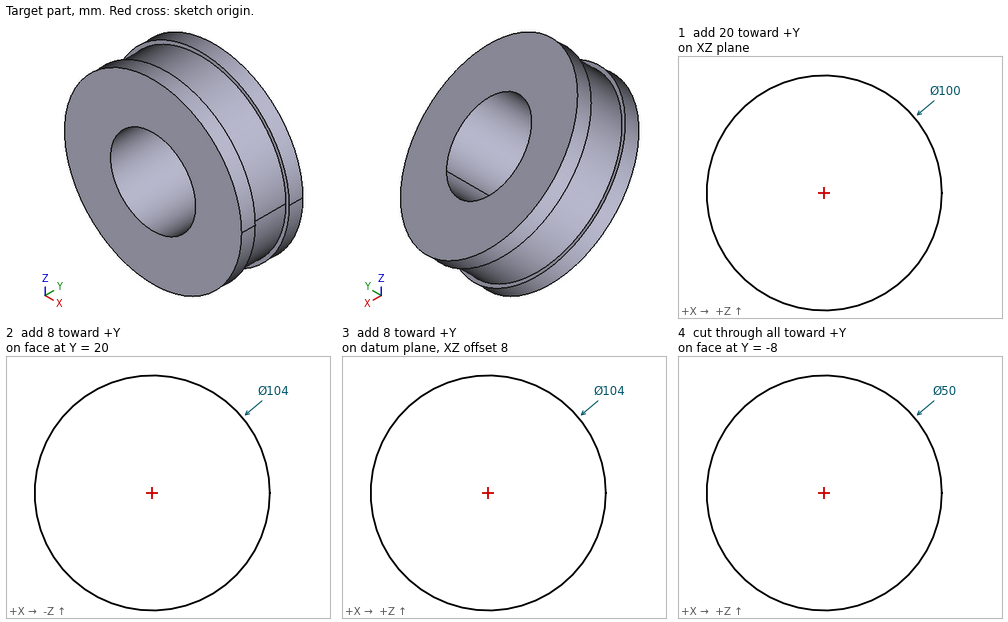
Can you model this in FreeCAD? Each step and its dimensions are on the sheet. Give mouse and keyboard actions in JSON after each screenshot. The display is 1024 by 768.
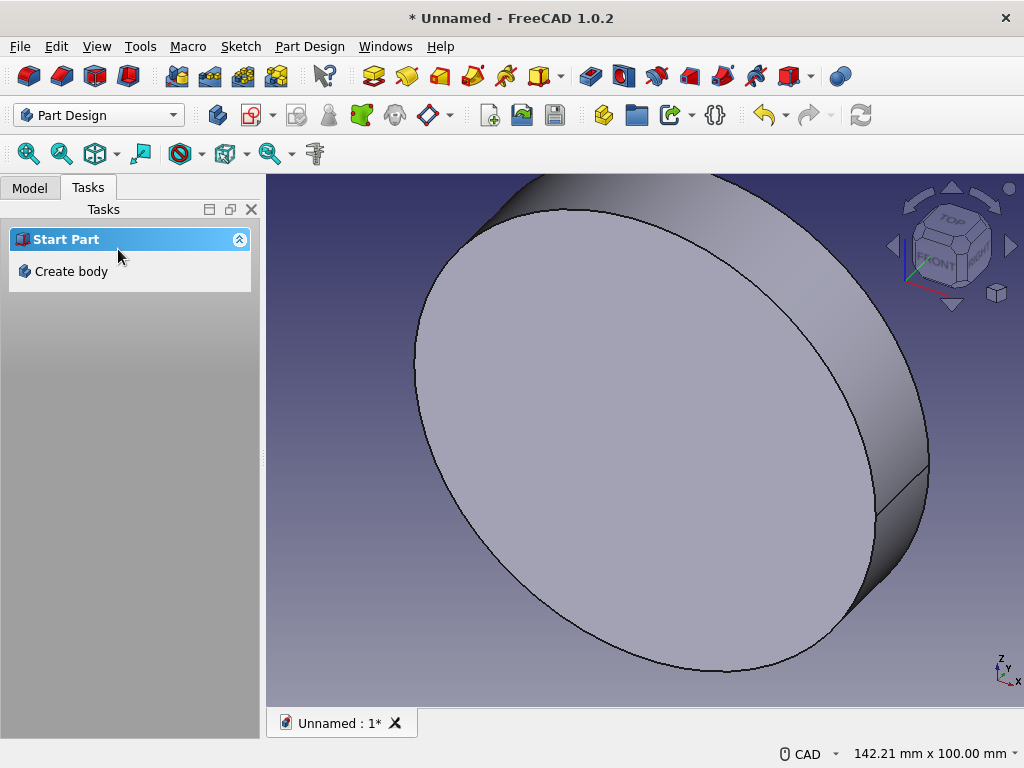
{"action": "left_click", "coordinate": [29, 154]}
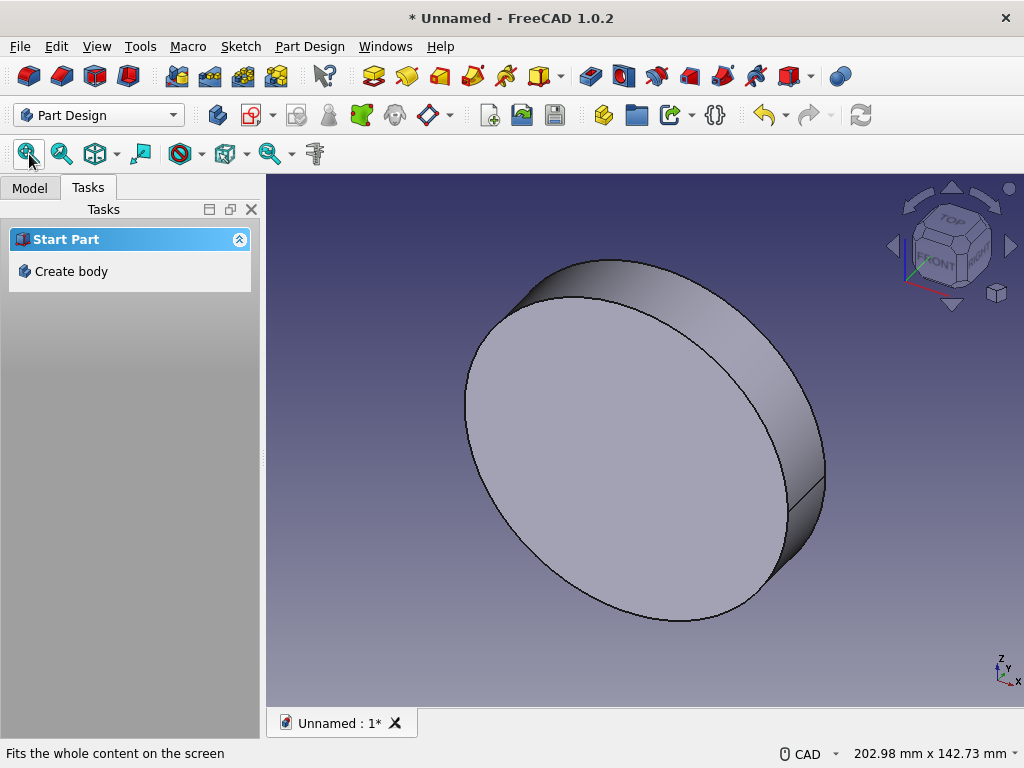
{"action": "key", "text": "4"}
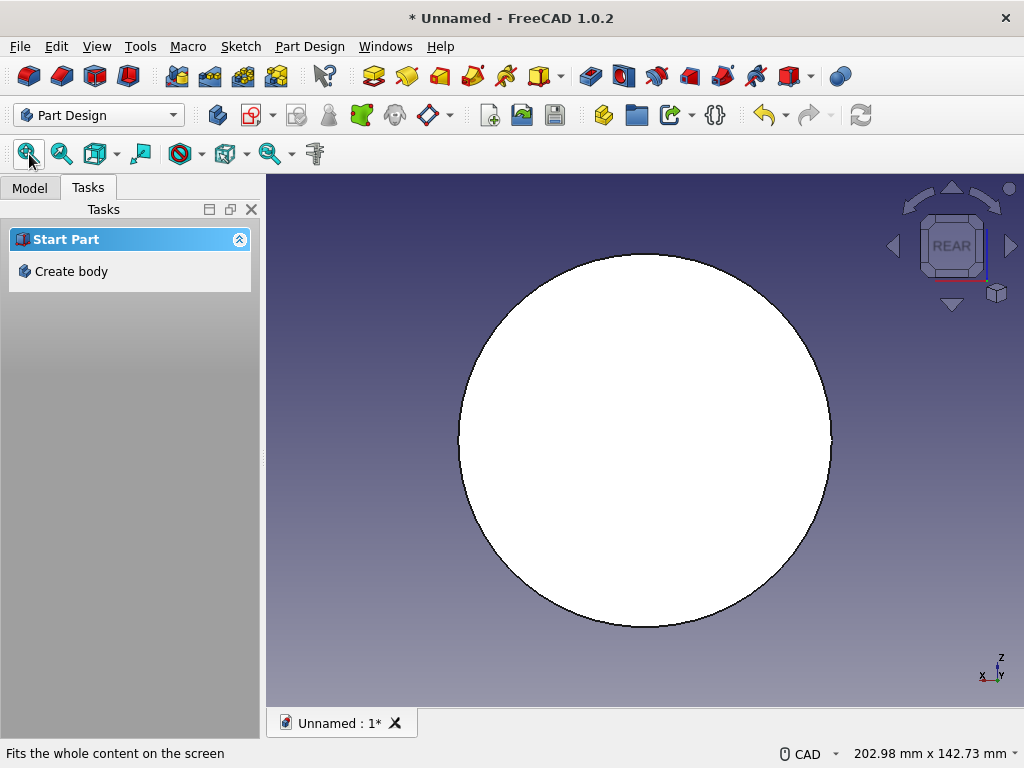
{"action": "left_click", "coordinate": [645, 440]}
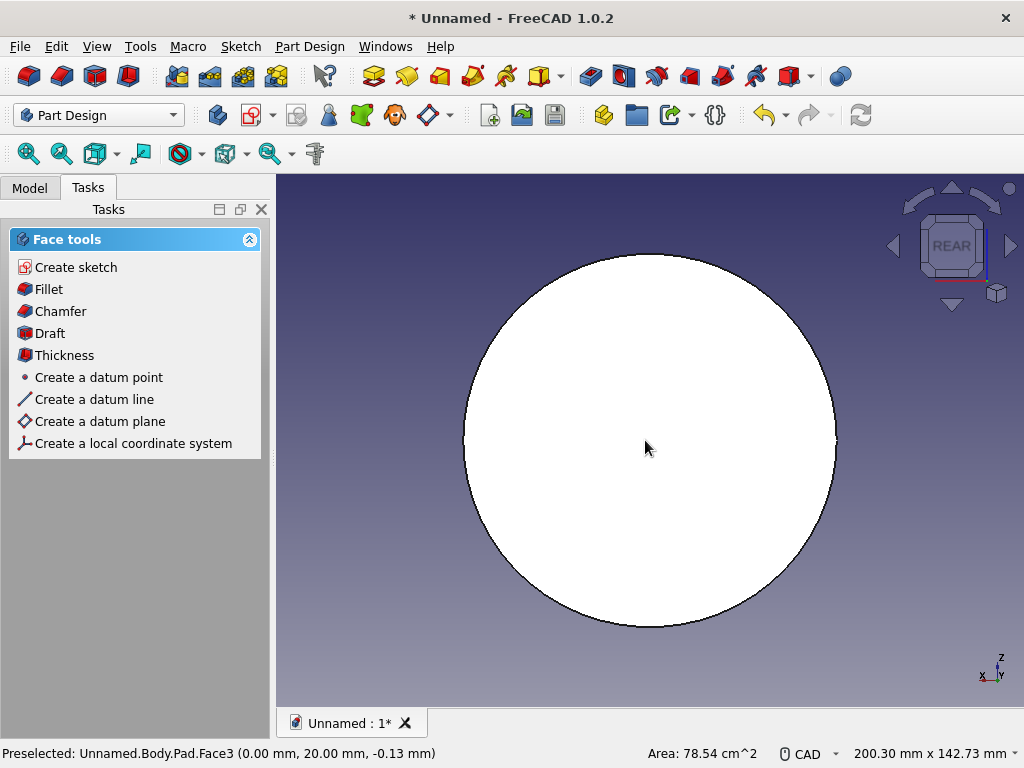
{"action": "left_click", "coordinate": [250, 116]}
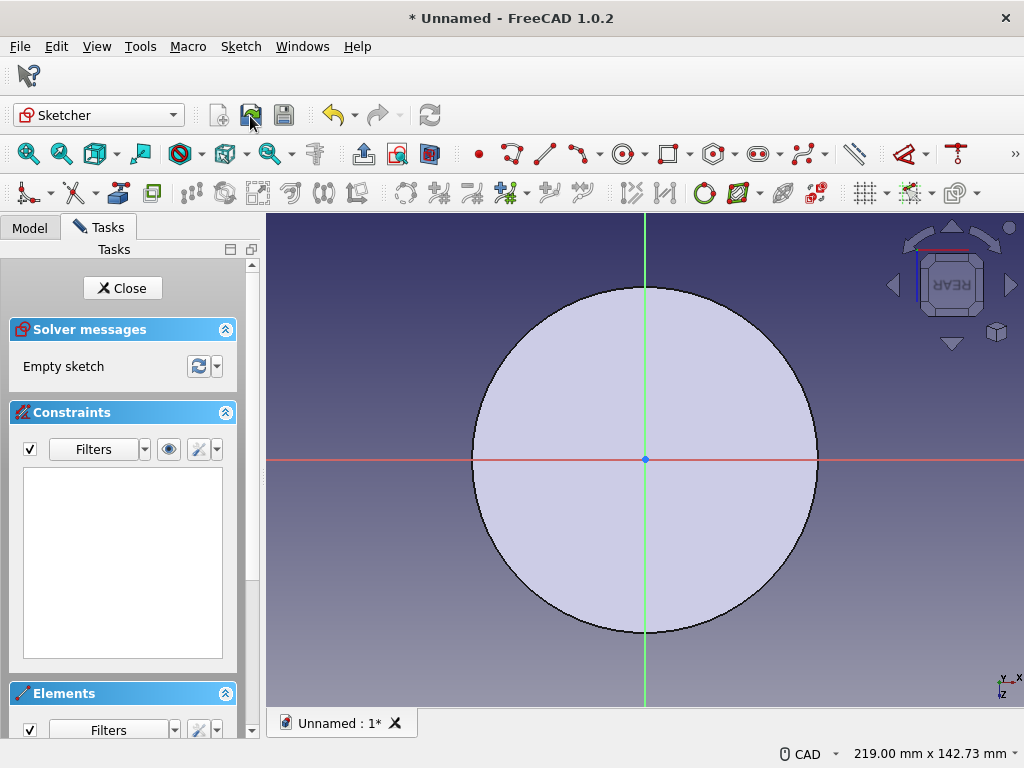
{"action": "left_click", "coordinate": [622, 154]}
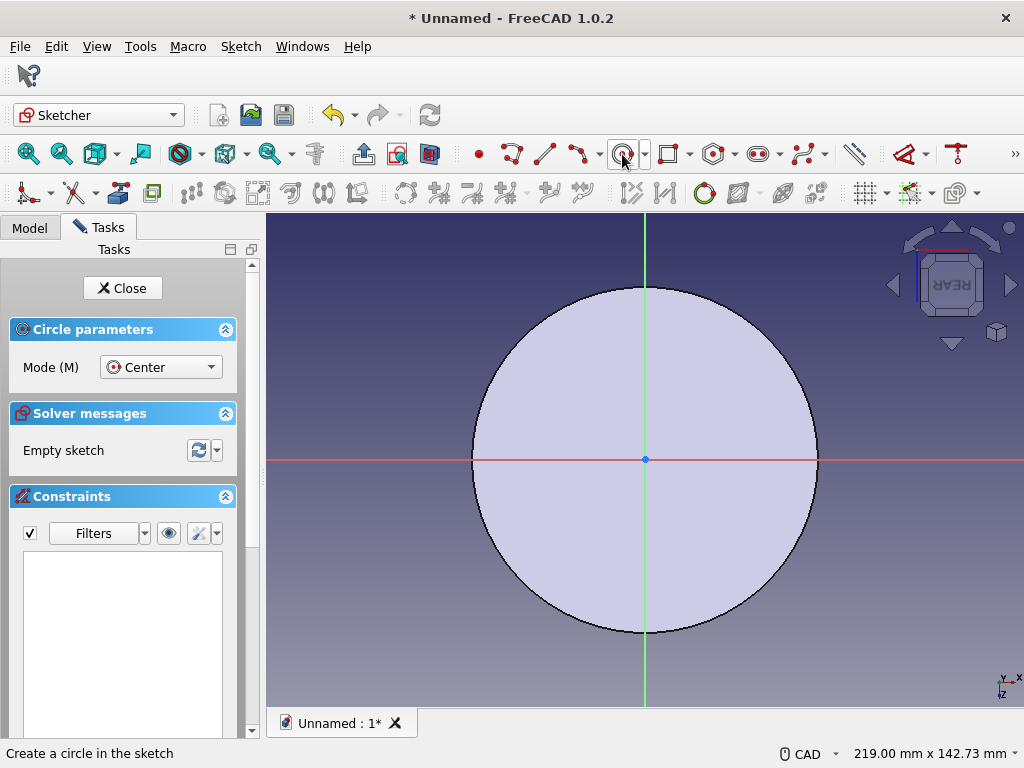
{"action": "left_click", "coordinate": [645, 460]}
{"action": "mouse_move", "coordinate": [772, 333]}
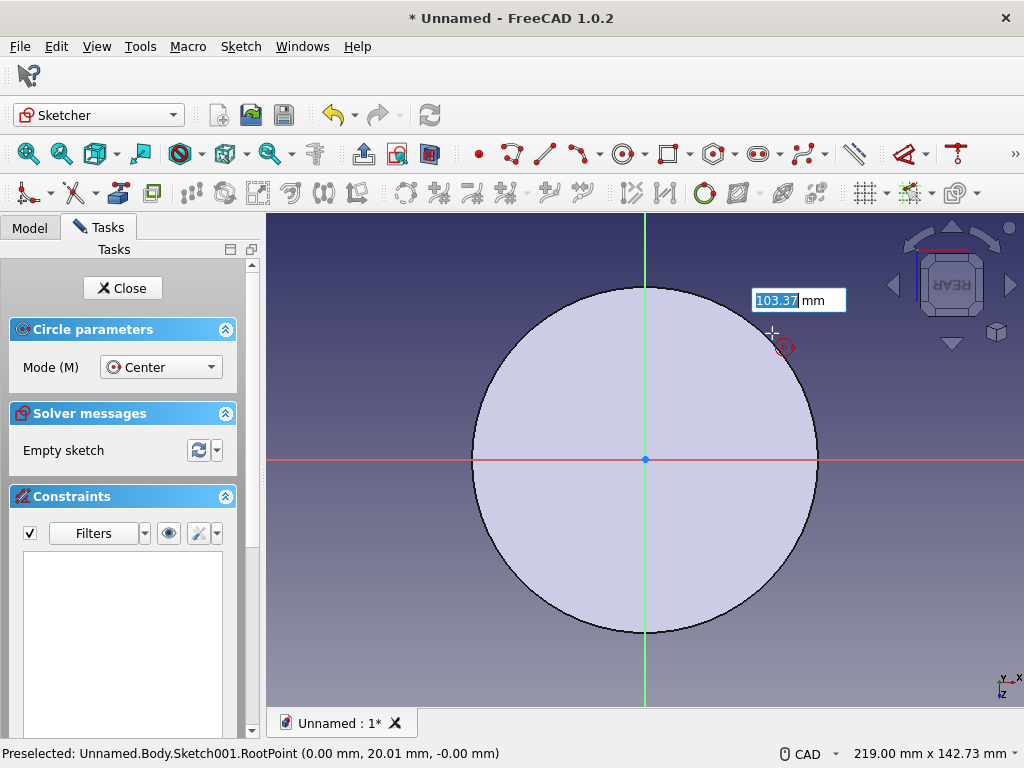
{"action": "type", "text": "104"}
{"action": "key", "text": "Return"}
{"action": "key", "text": "Escape"}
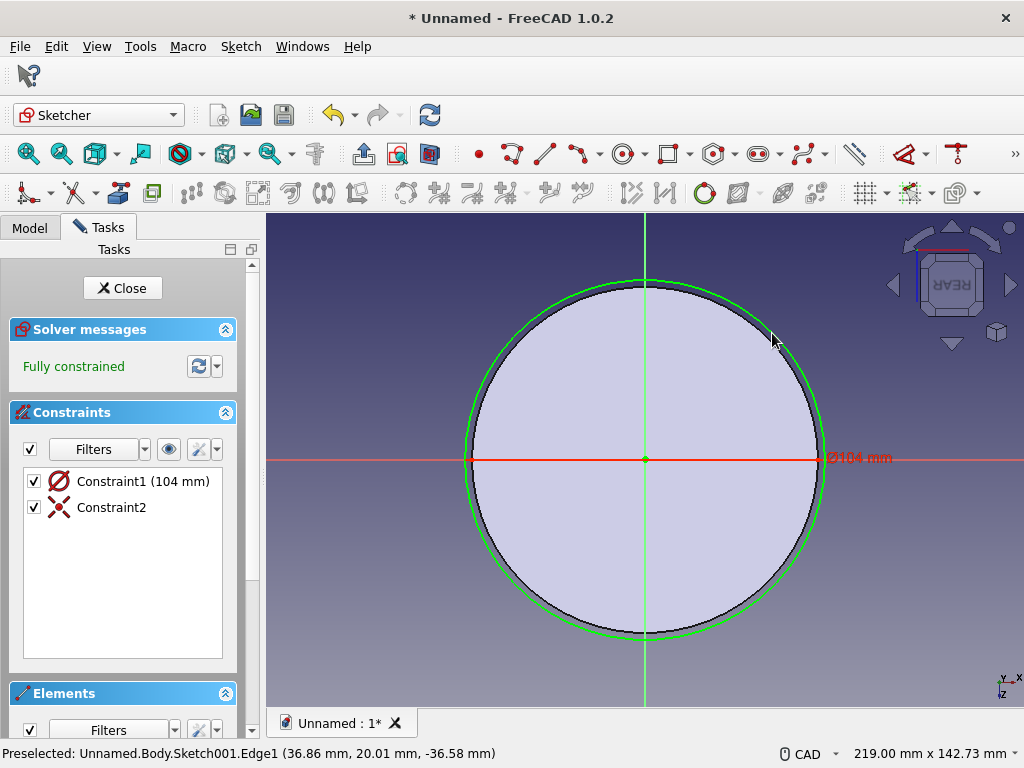
{"action": "left_click", "coordinate": [123, 288]}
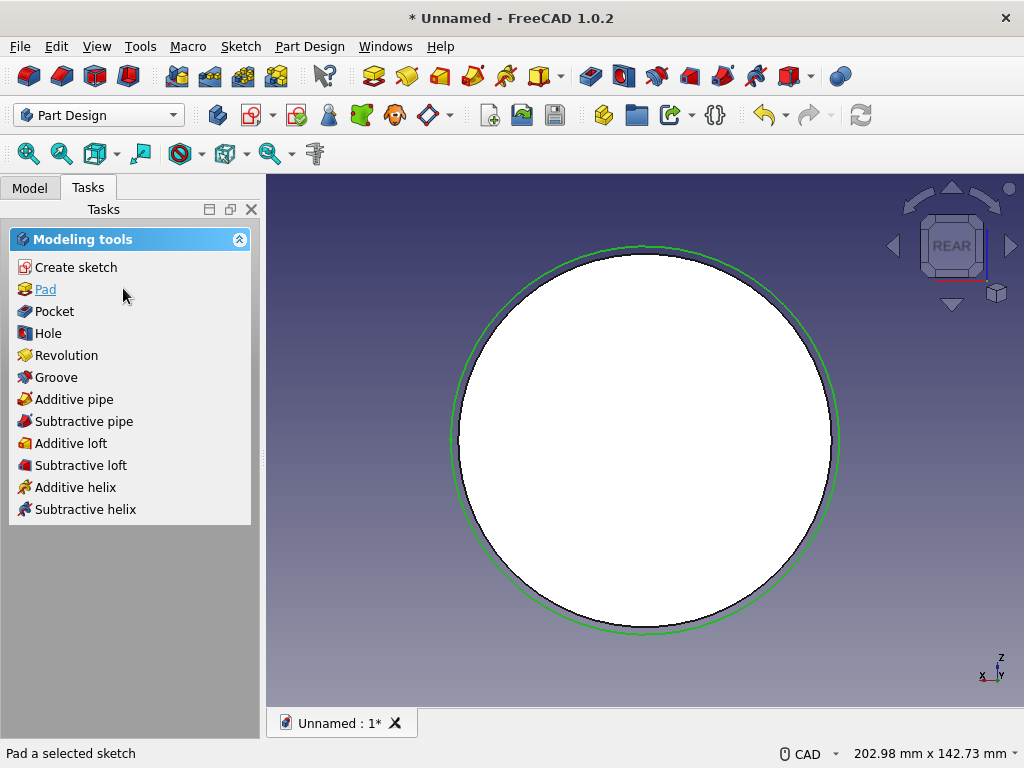
{"action": "left_click", "coordinate": [374, 76]}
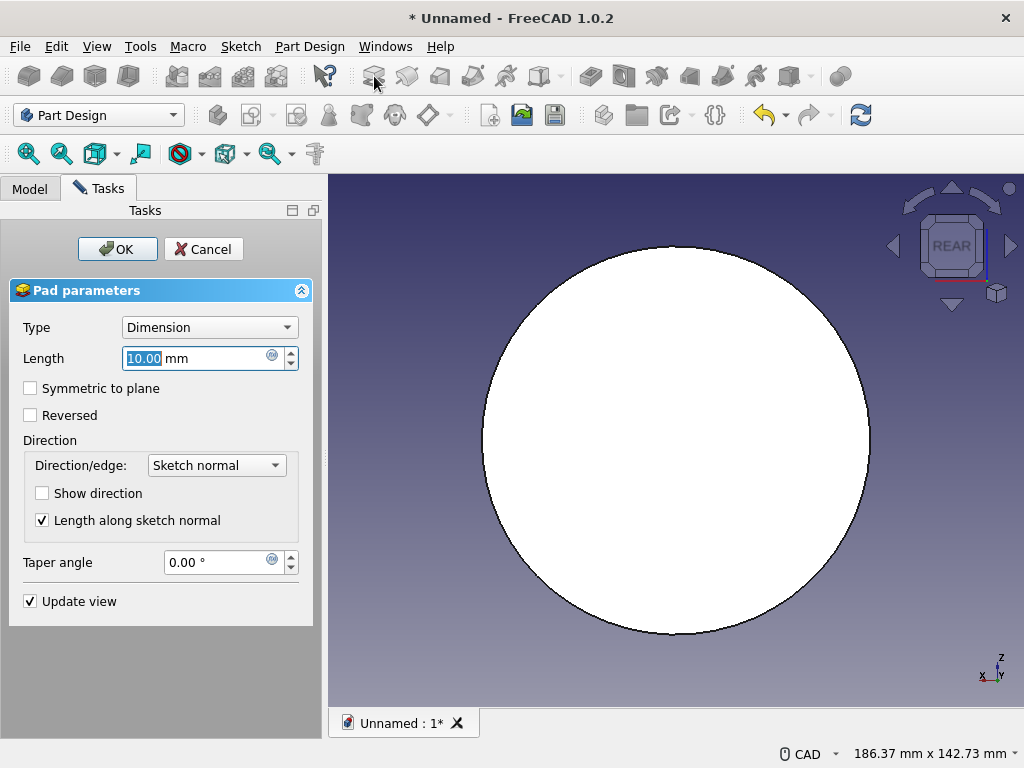
{"action": "type", "text": "8"}
{"action": "key", "text": "Tab"}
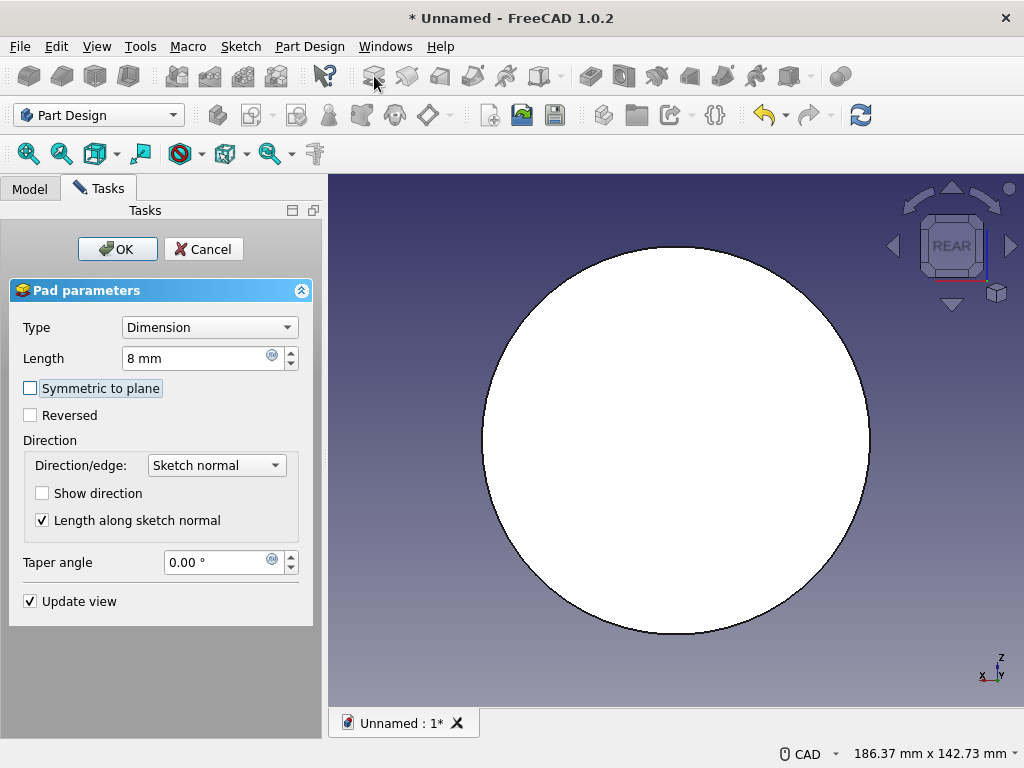
{"action": "left_click", "coordinate": [118, 249]}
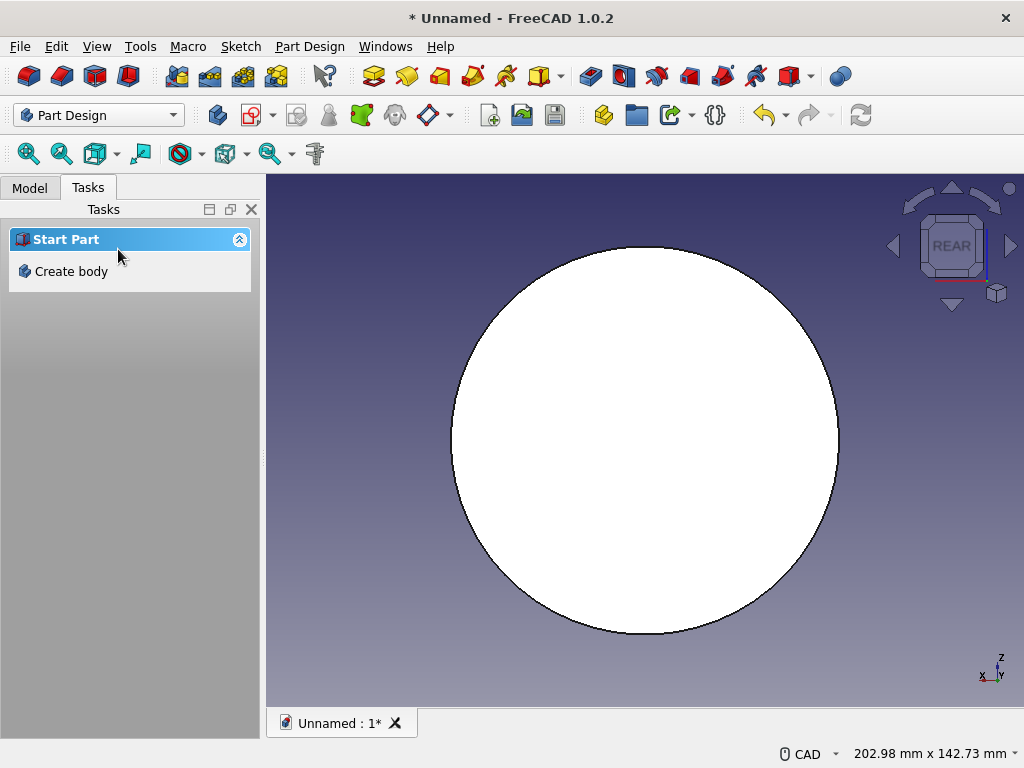
{"action": "left_click", "coordinate": [30, 188]}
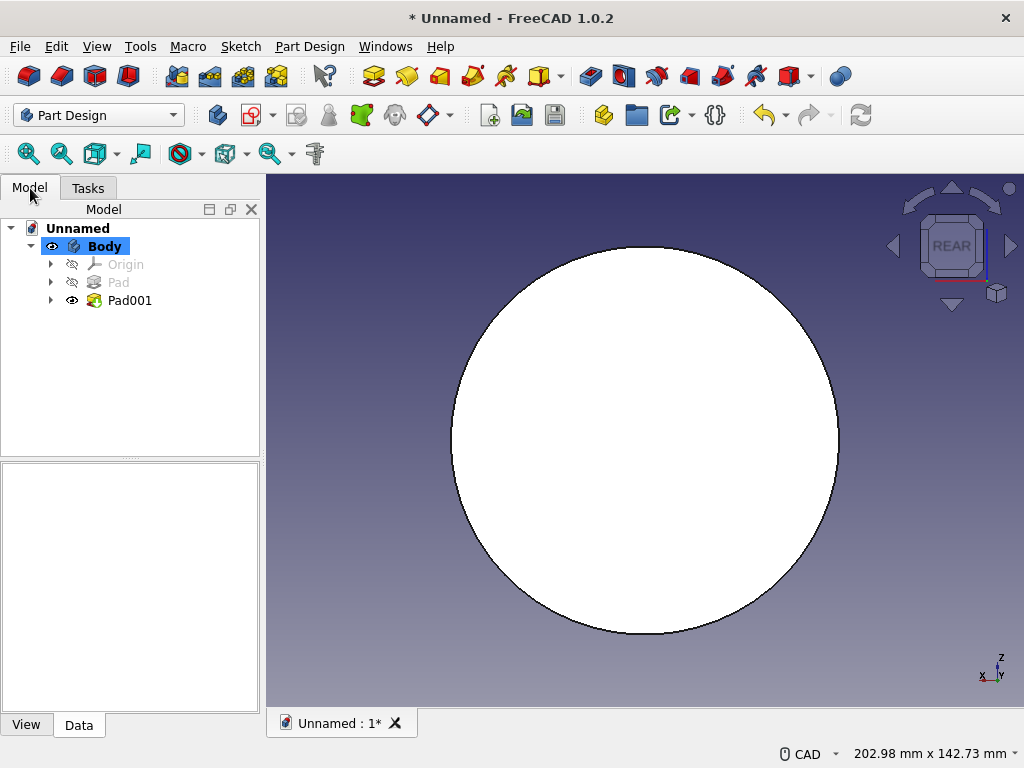
{"action": "left_click", "coordinate": [51, 264]}